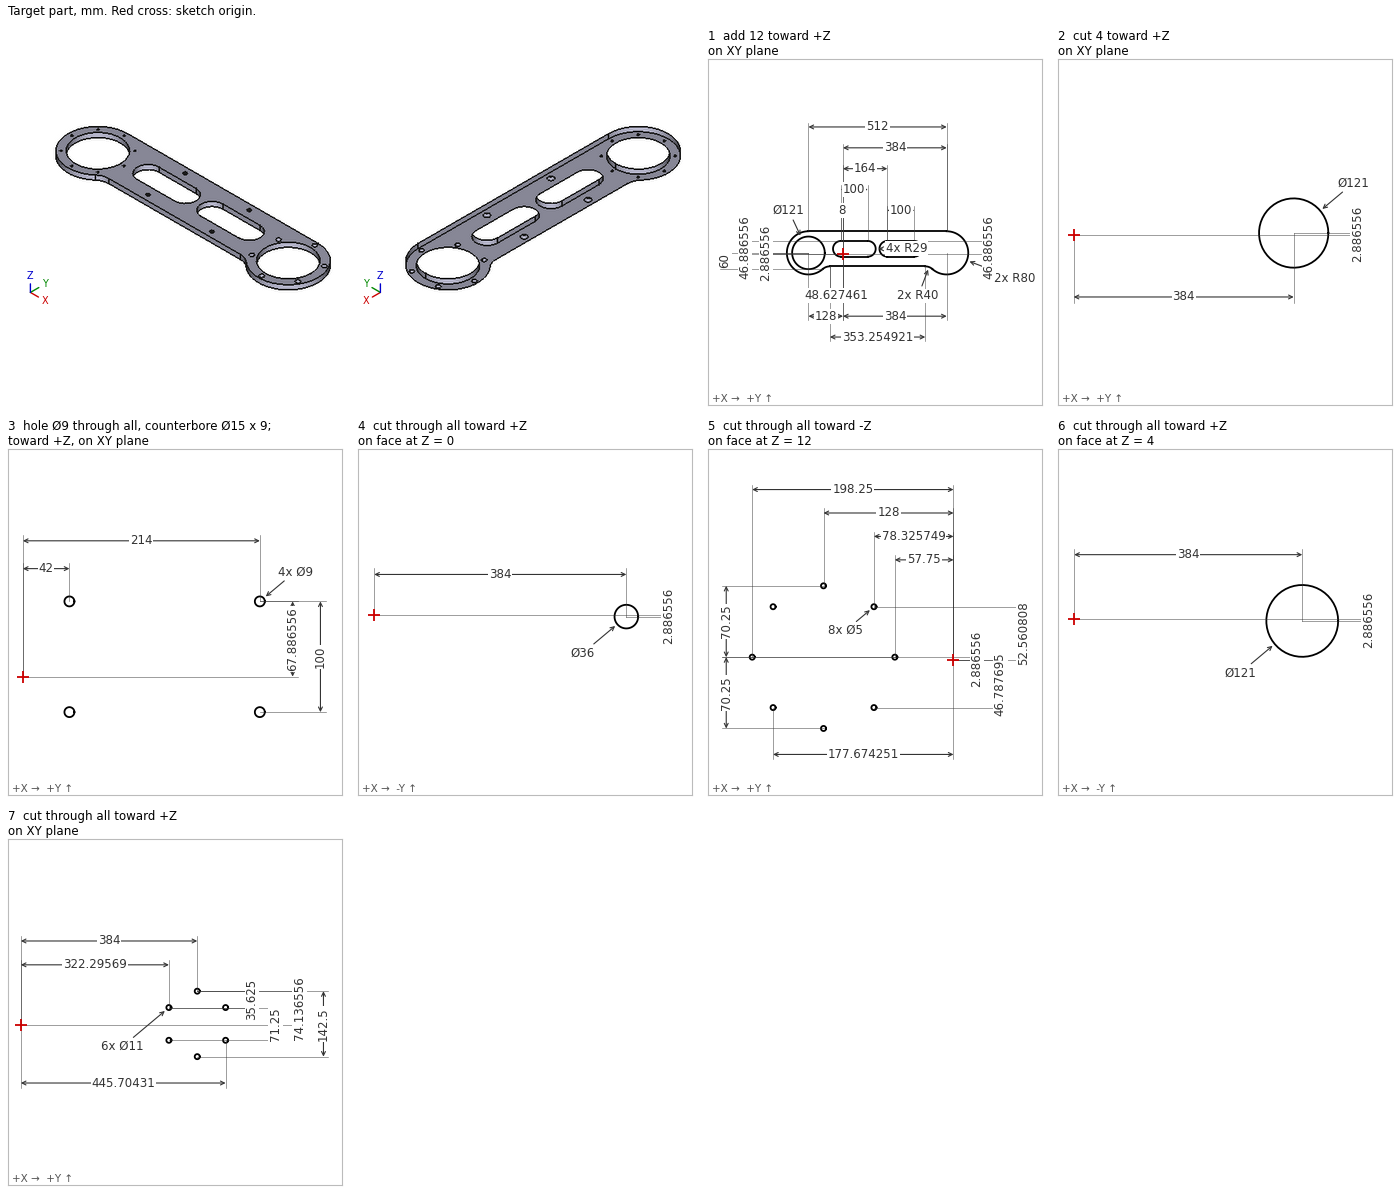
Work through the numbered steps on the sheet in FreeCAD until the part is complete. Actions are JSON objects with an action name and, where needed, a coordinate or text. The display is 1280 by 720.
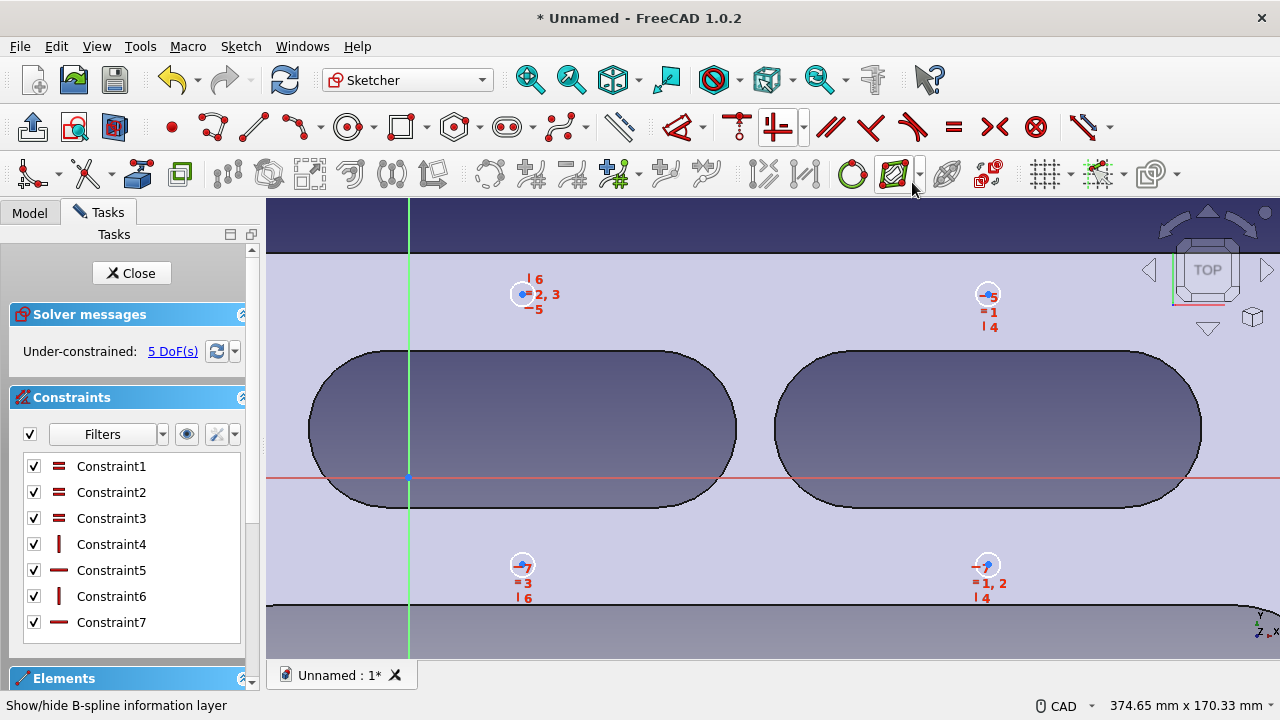
{"action": "left_click", "coordinate": [676, 128]}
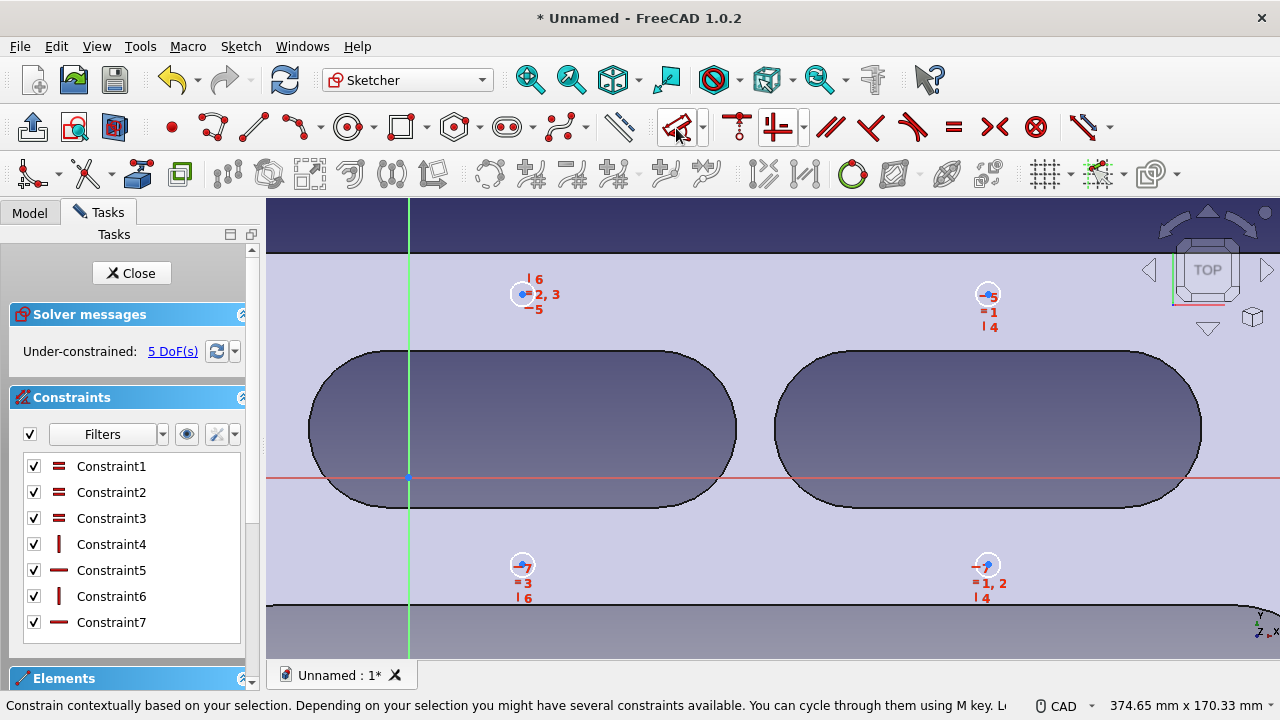
{"action": "scroll", "coordinate": [997, 286], "scroll_direction": "up", "scroll_amount": 3}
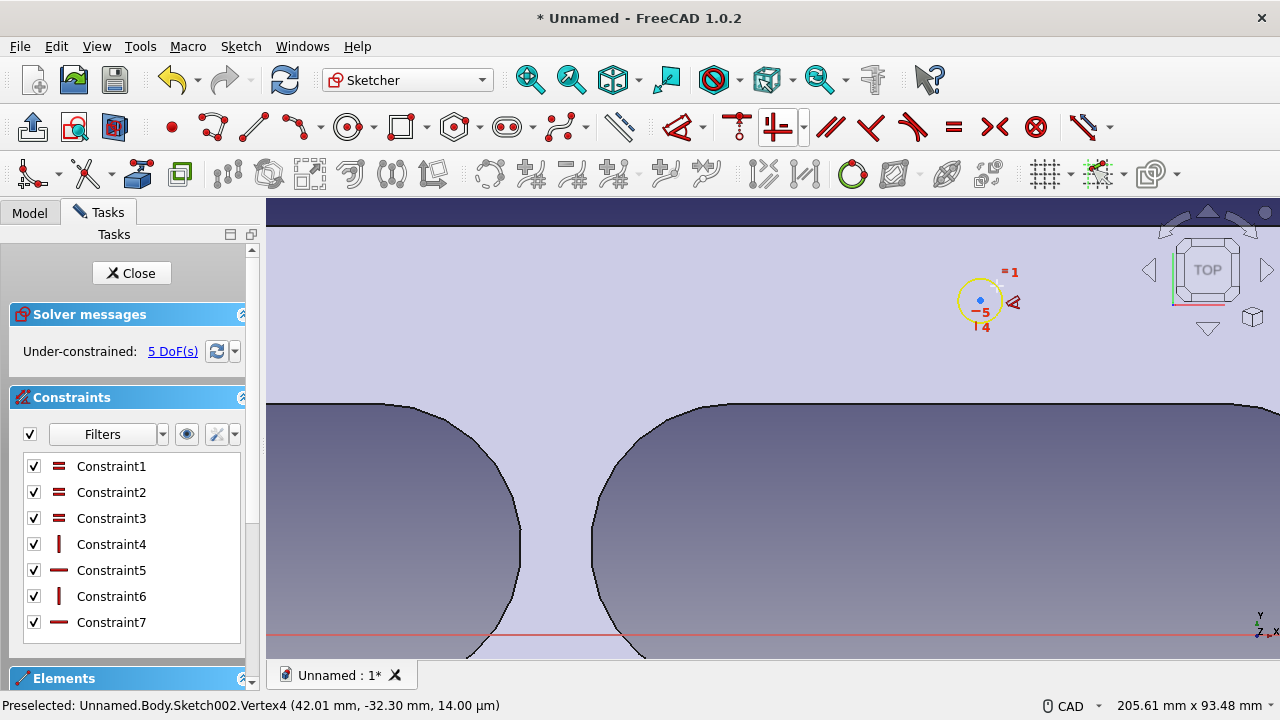
{"action": "left_click", "coordinate": [996, 285]}
{"action": "left_click", "coordinate": [1019, 262]}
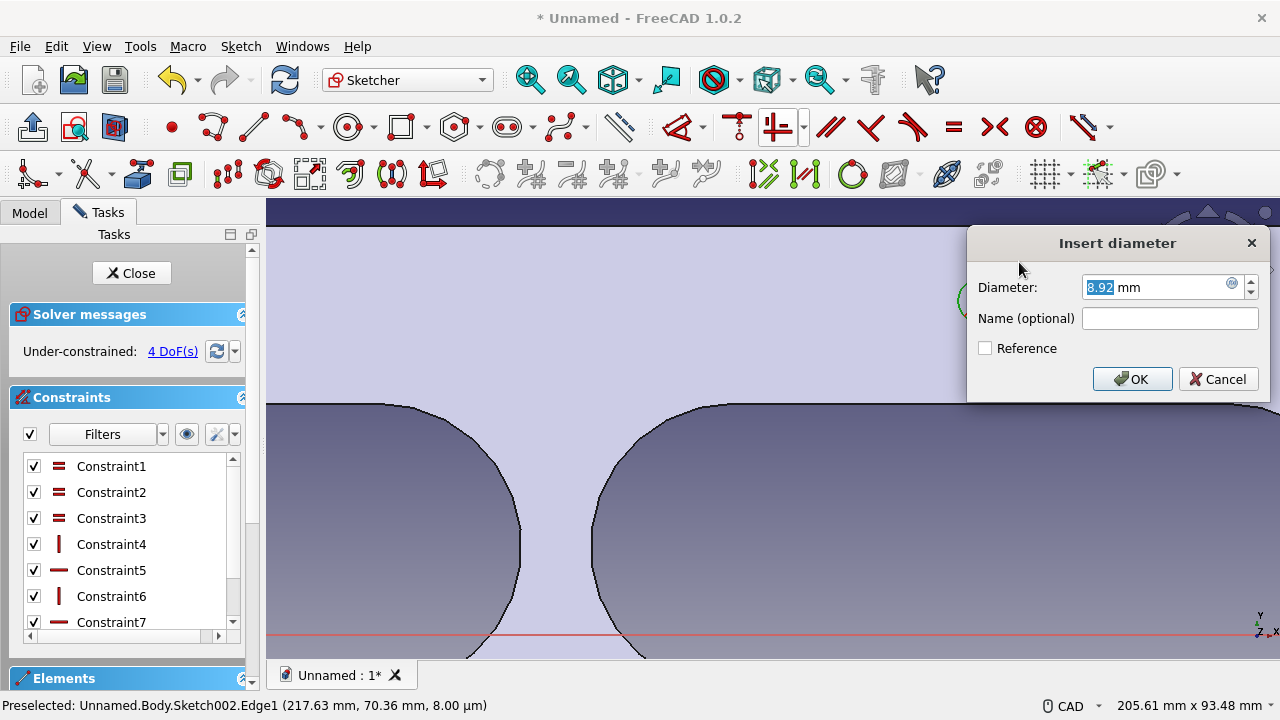
{"action": "type", "text": "9"}
{"action": "key", "text": "Return"}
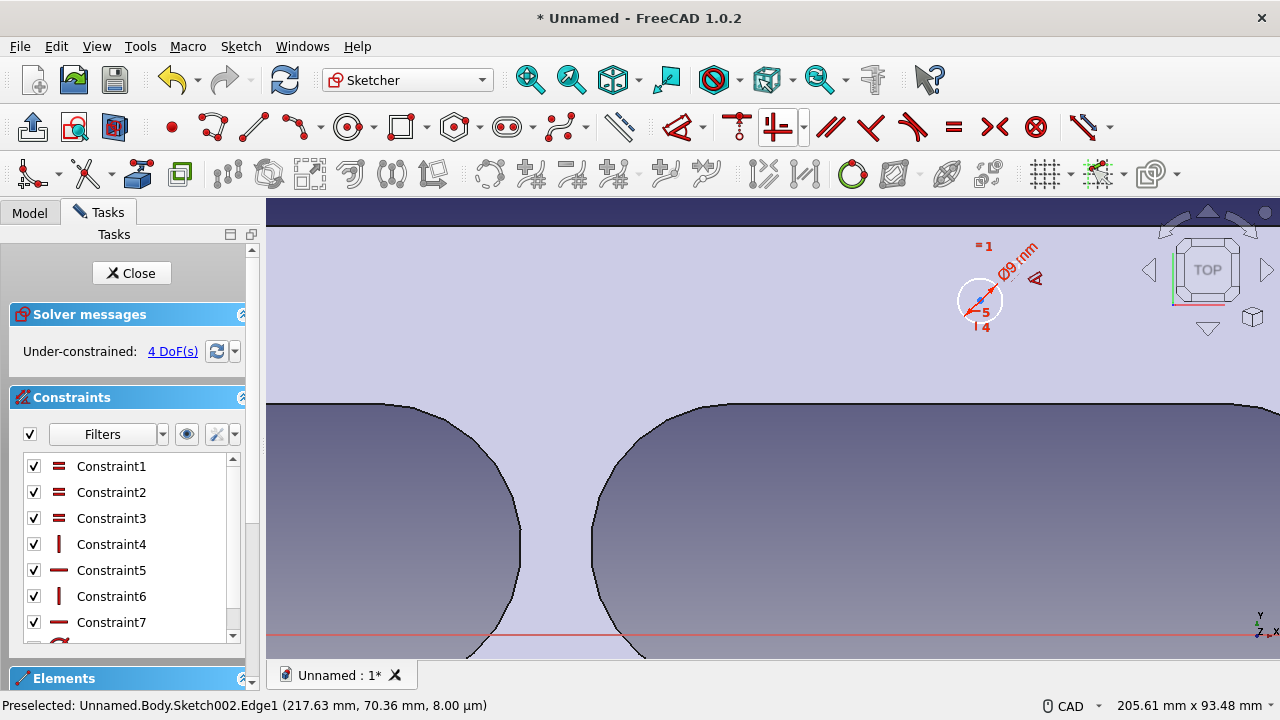
{"action": "scroll", "coordinate": [998, 285], "scroll_direction": "down", "scroll_amount": 3}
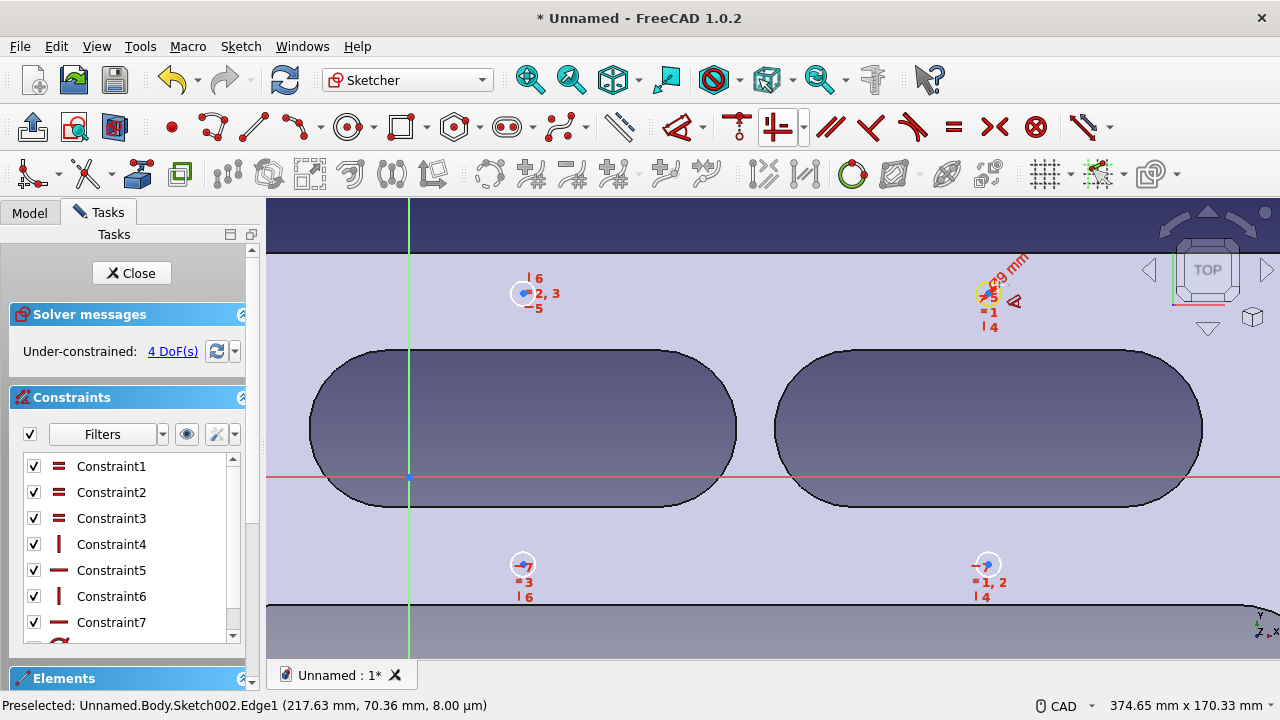
{"action": "left_click", "coordinate": [523, 294]}
{"action": "left_click", "coordinate": [466, 260]}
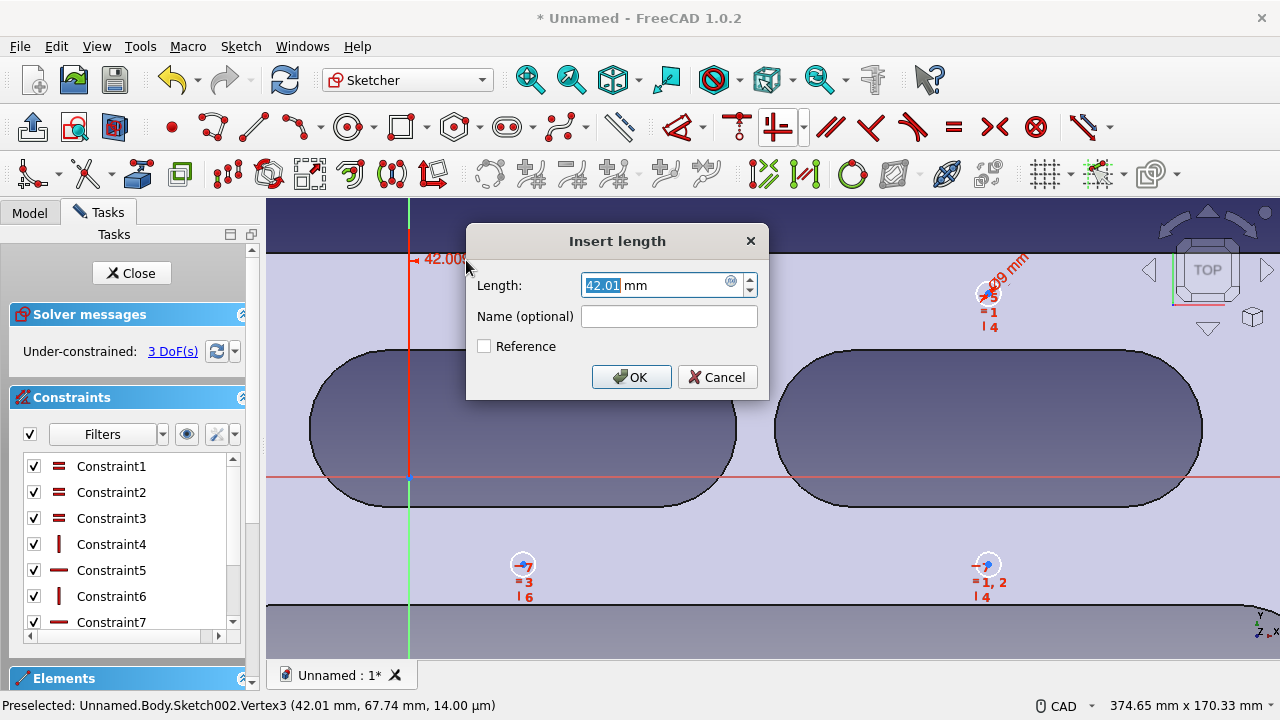
{"action": "type", "text": "42"}
{"action": "key", "text": "Return"}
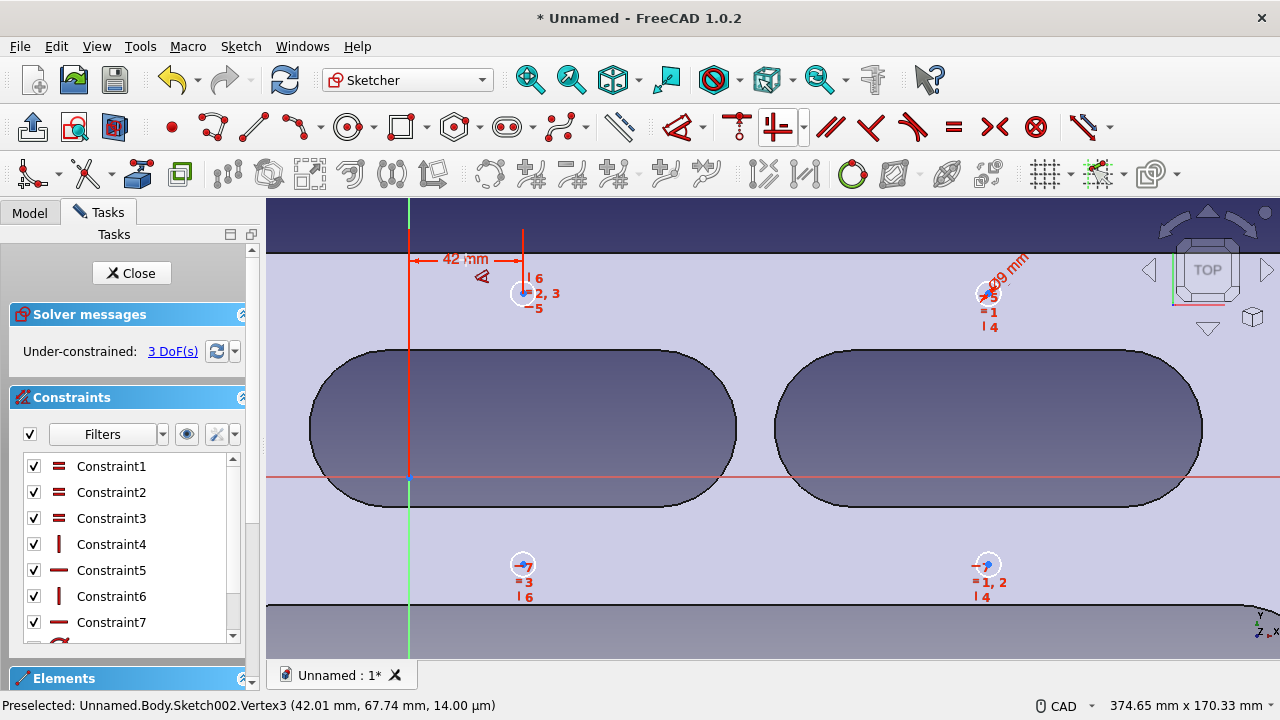
{"action": "left_click", "coordinate": [989, 294]}
{"action": "left_click", "coordinate": [699, 260]}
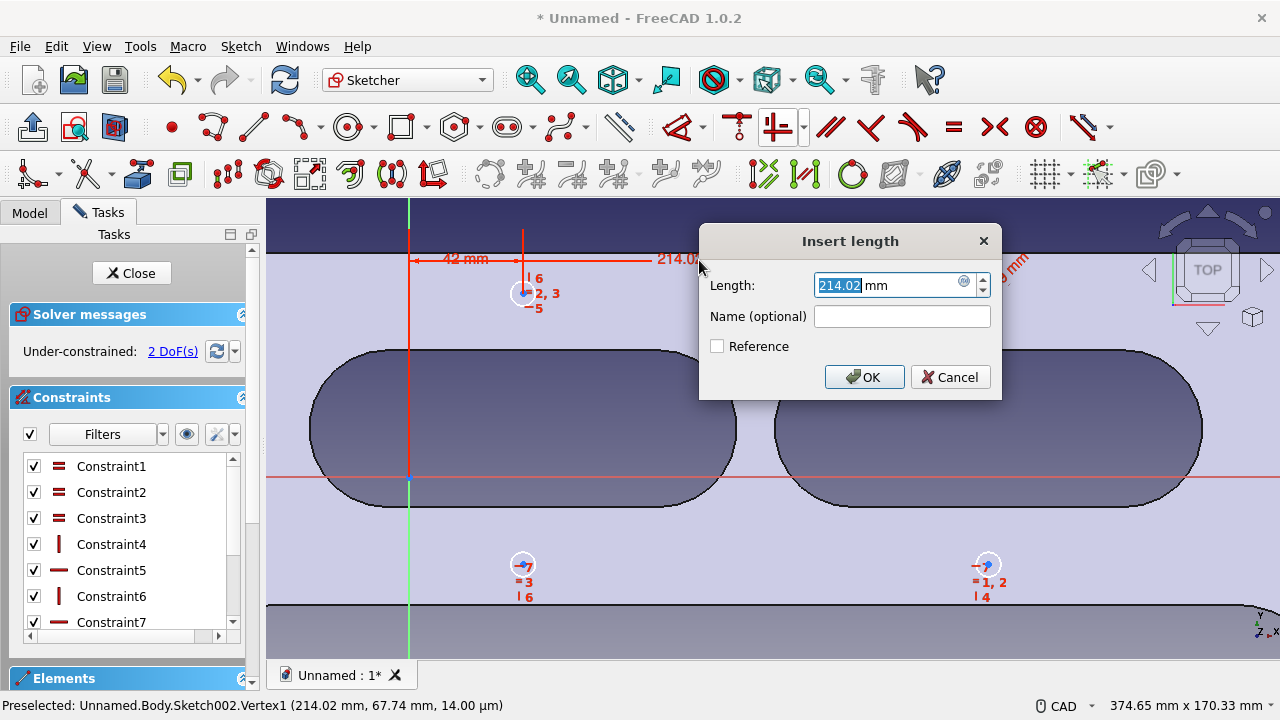
{"action": "type", "text": "214"}
{"action": "key", "text": "Return"}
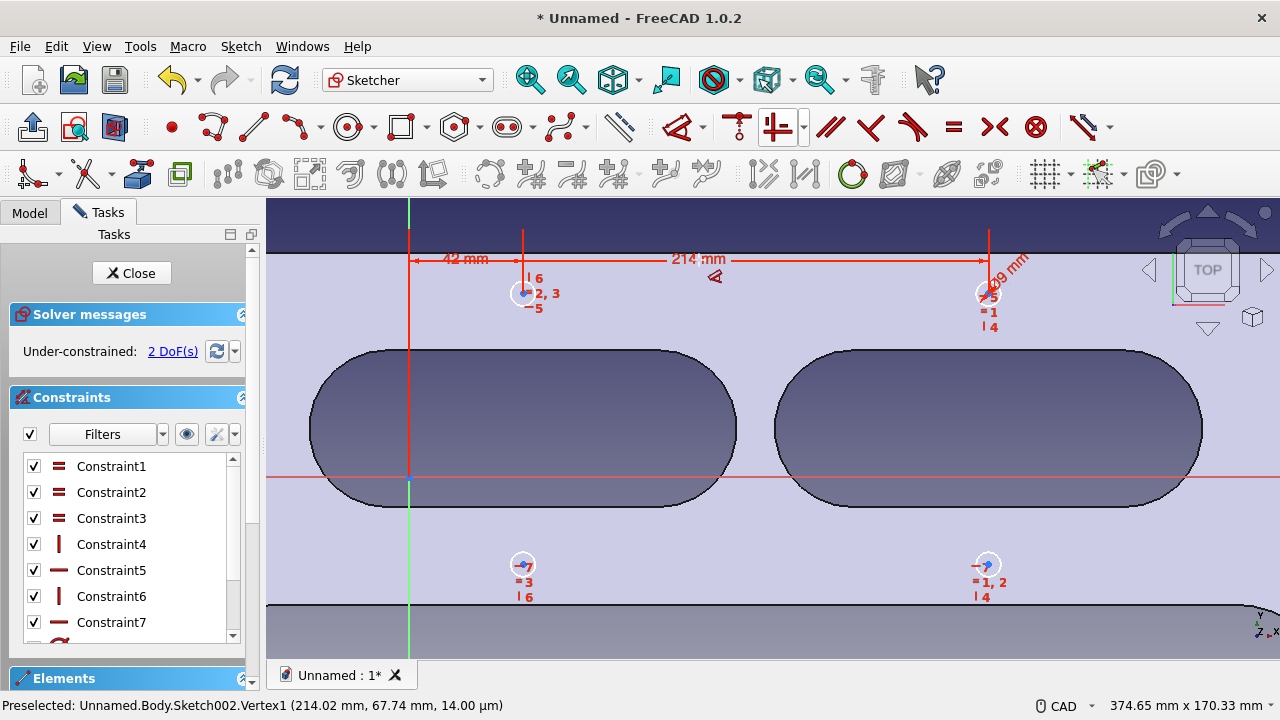
{"action": "left_click", "coordinate": [989, 294]}